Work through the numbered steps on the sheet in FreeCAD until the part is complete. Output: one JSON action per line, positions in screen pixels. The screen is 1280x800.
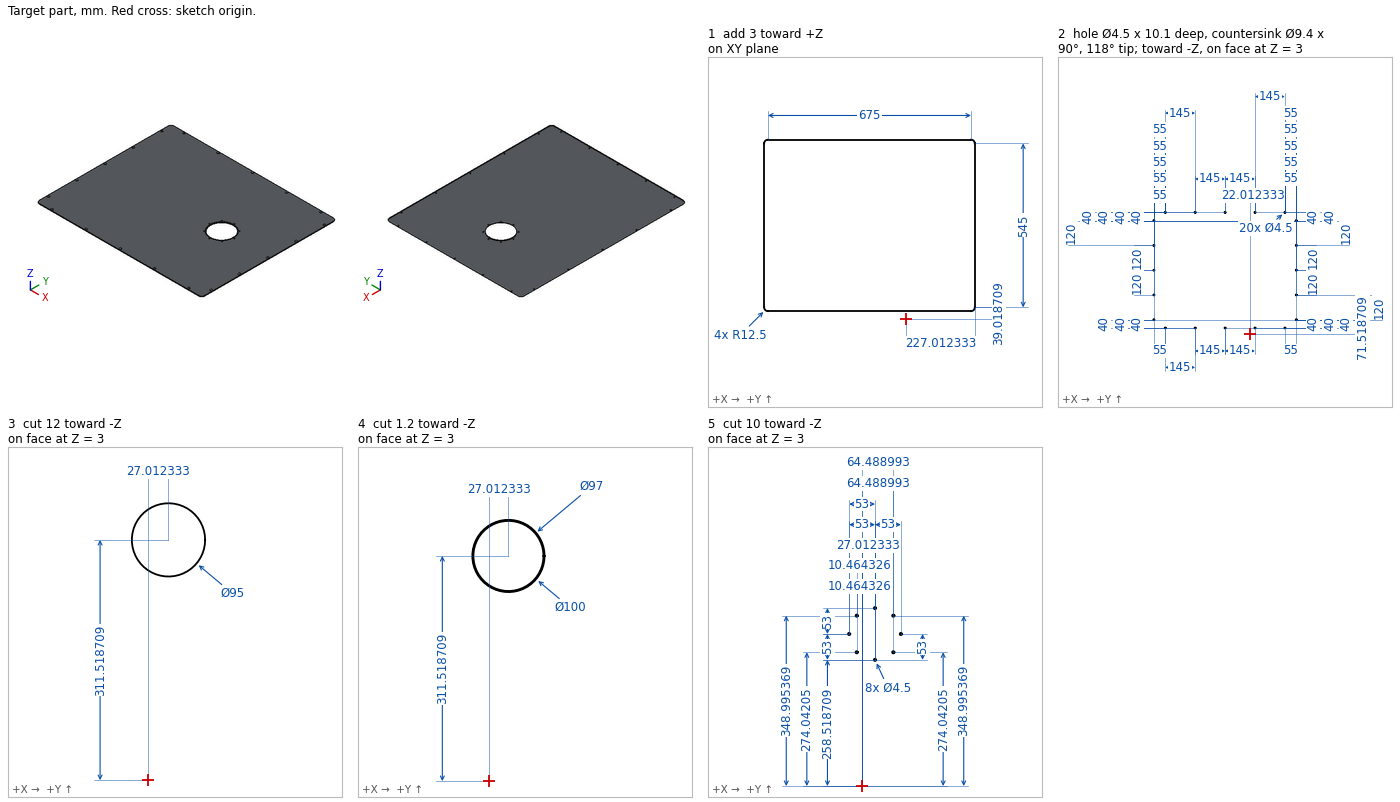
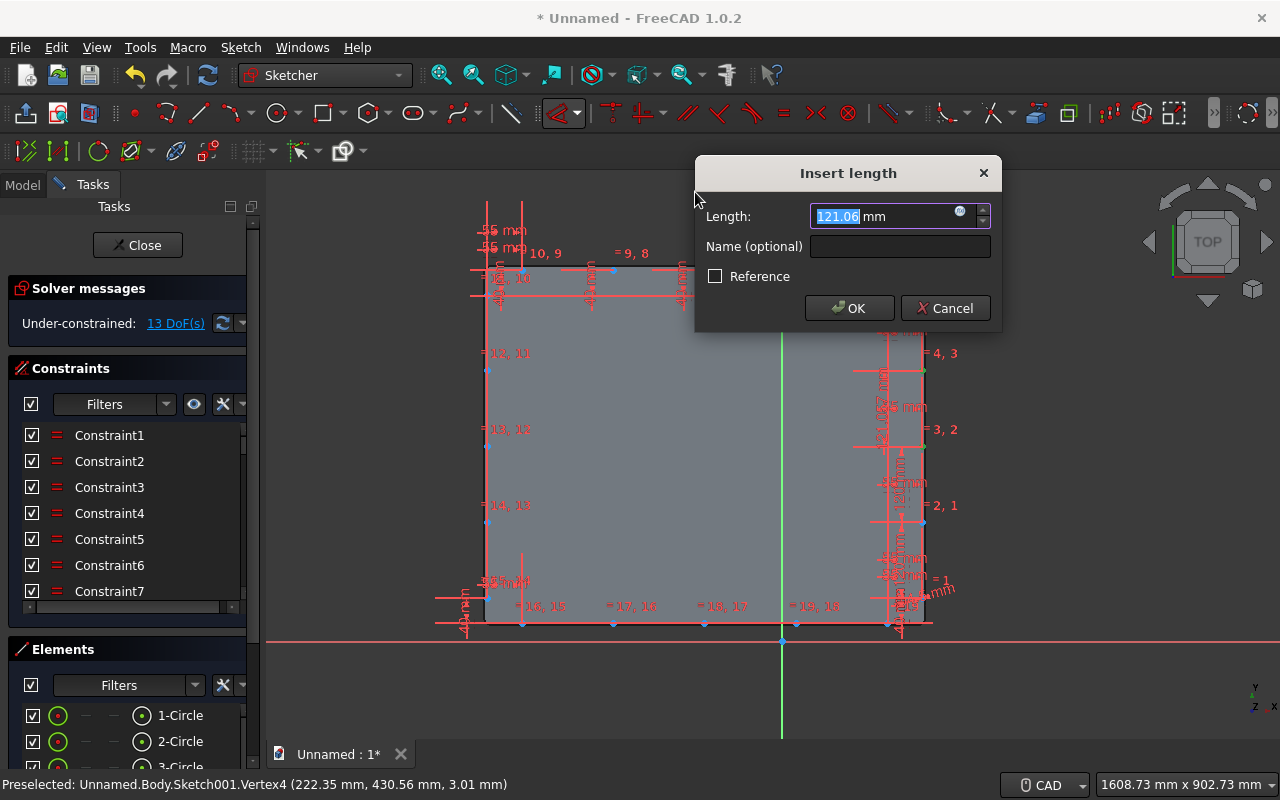
{"action": "type", "text": "120"}
{"action": "key", "text": "Return"}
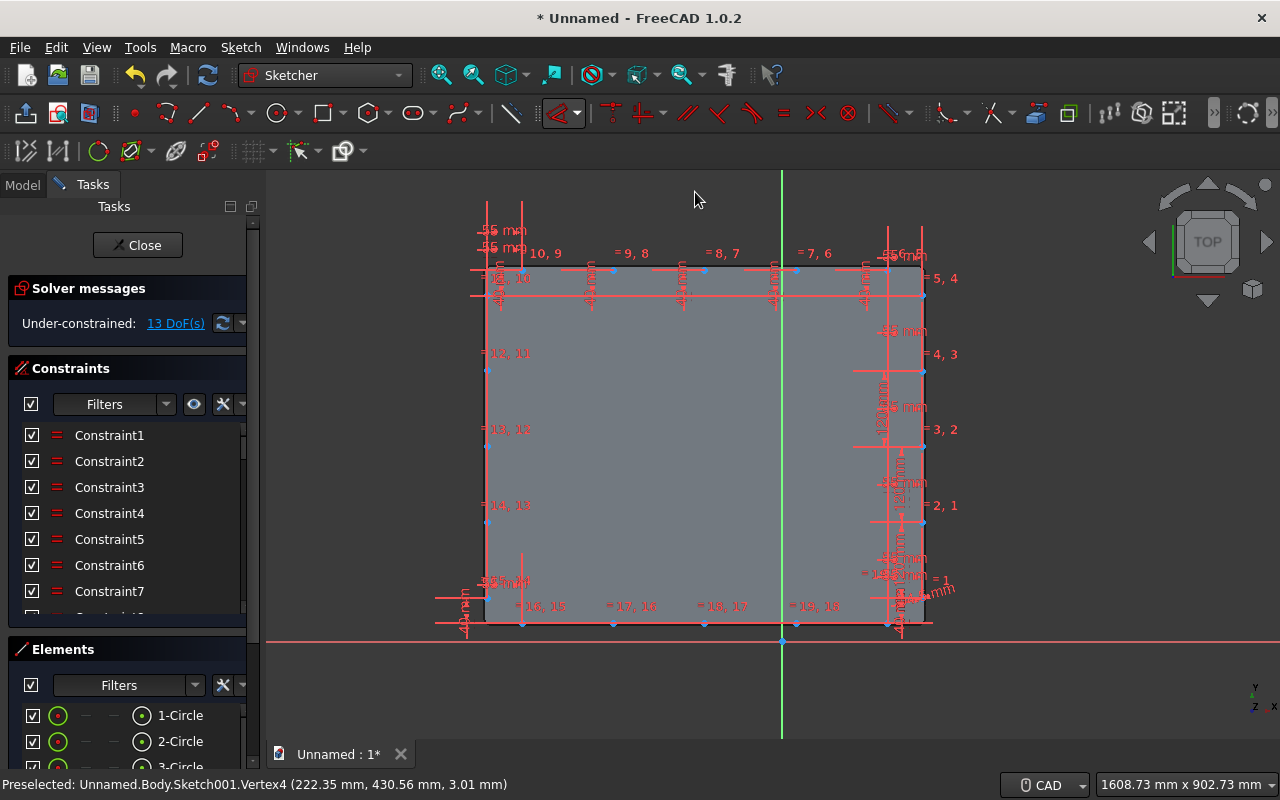
{"action": "left_click", "coordinate": [922, 371]}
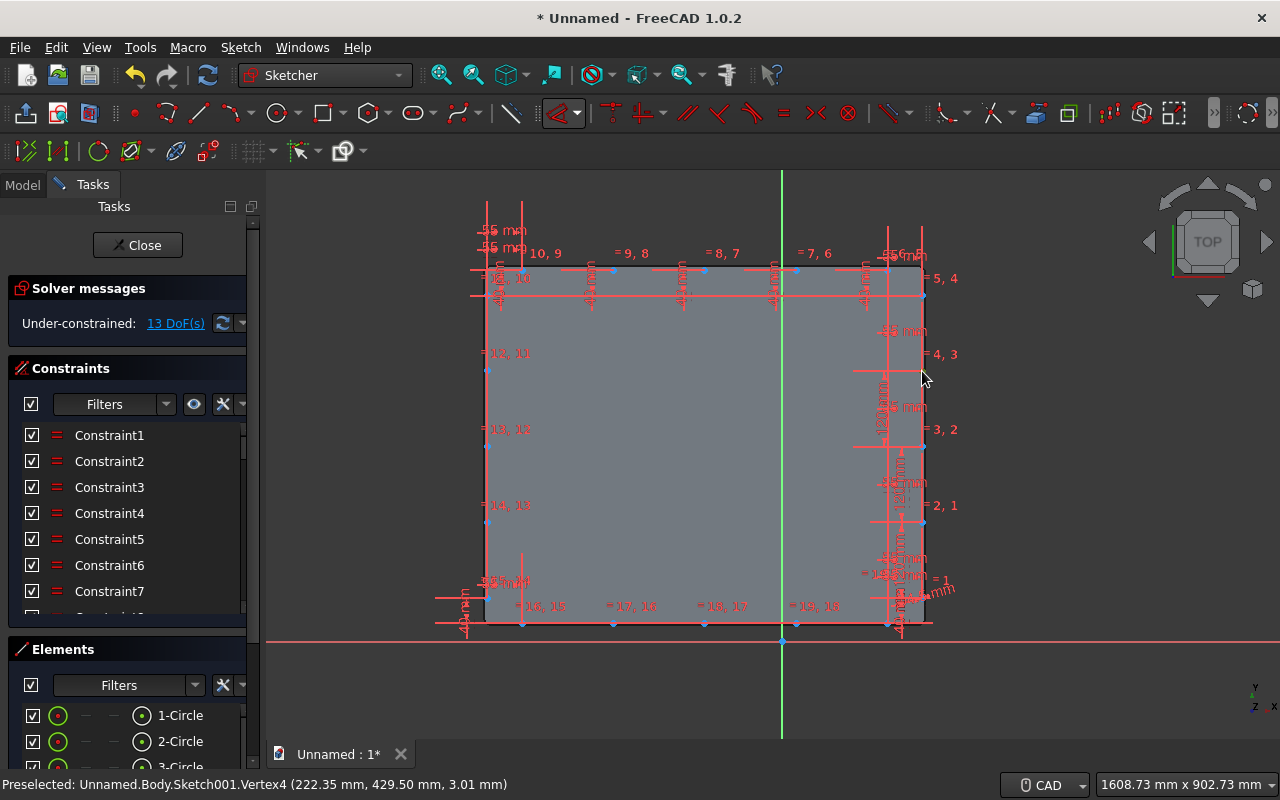
{"action": "left_click", "coordinate": [922, 296]}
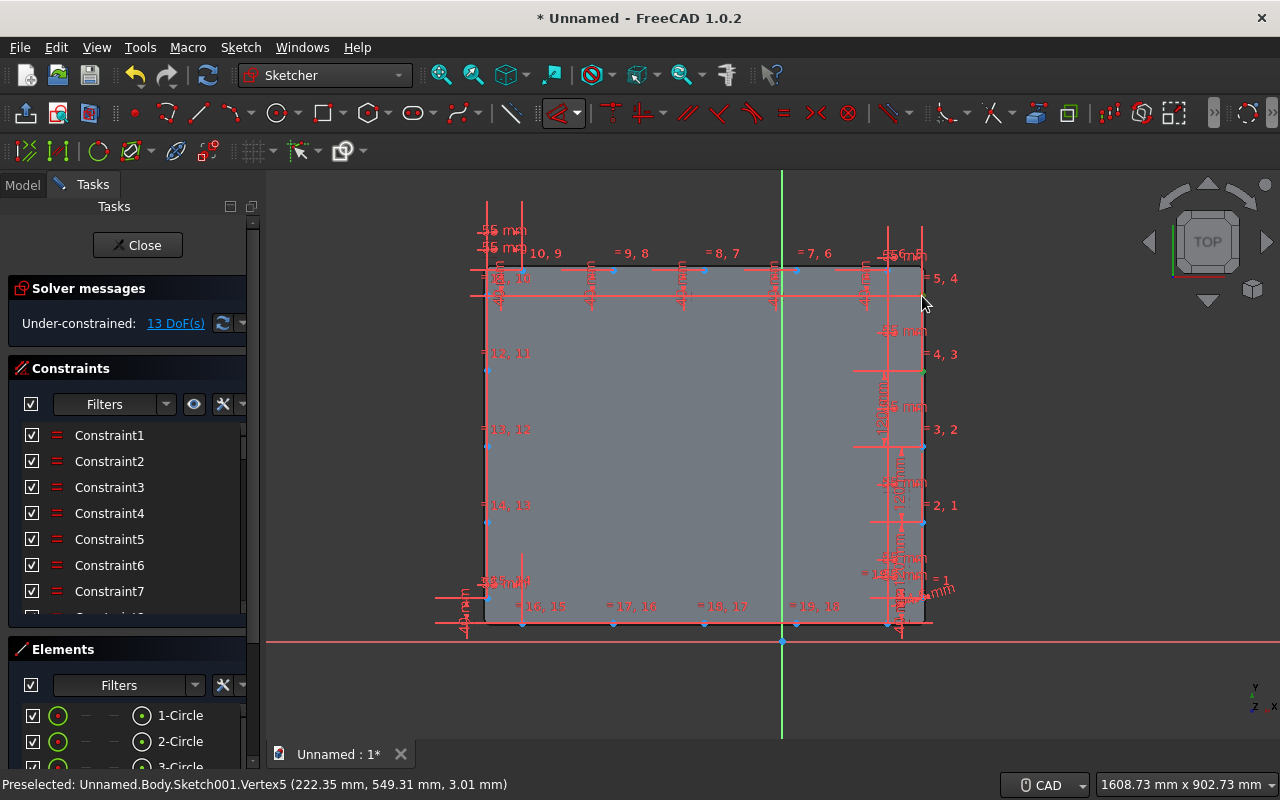
{"action": "key", "text": "i"}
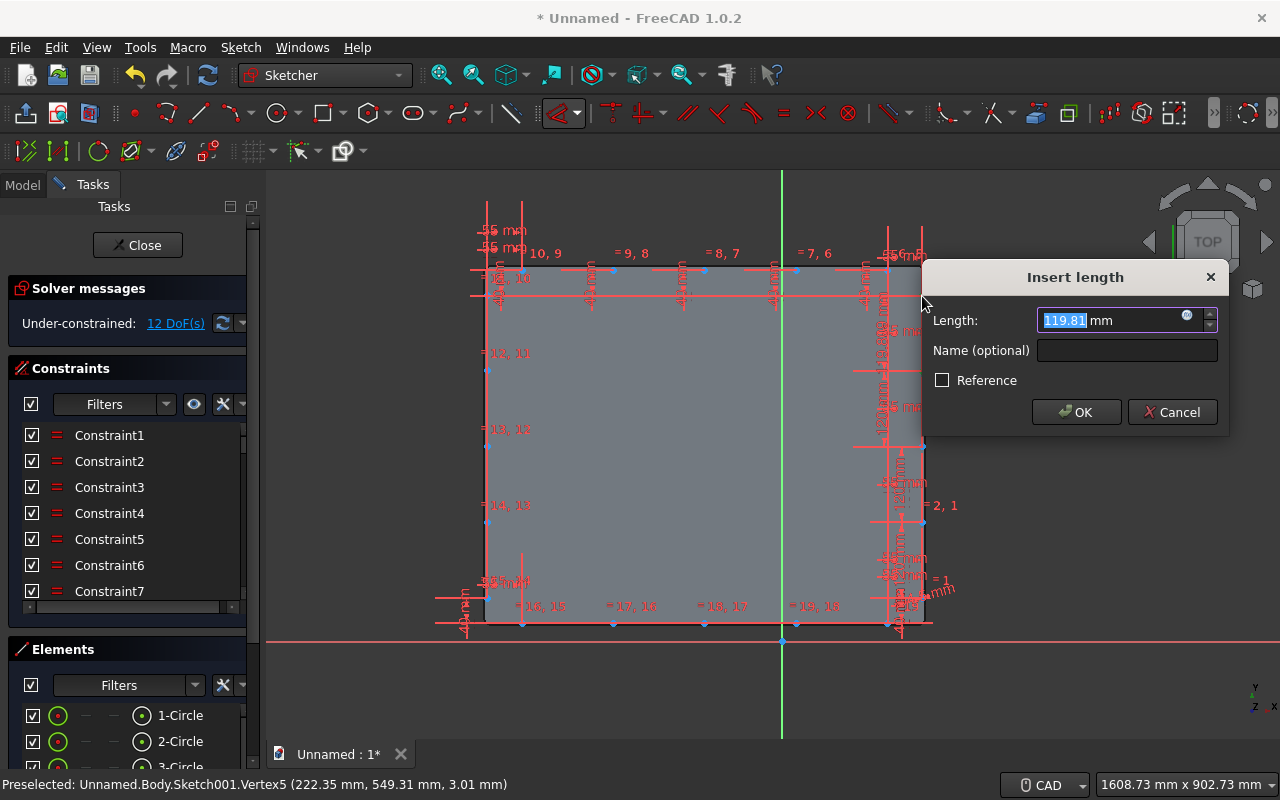
{"action": "type", "text": "120"}
{"action": "key", "text": "Return"}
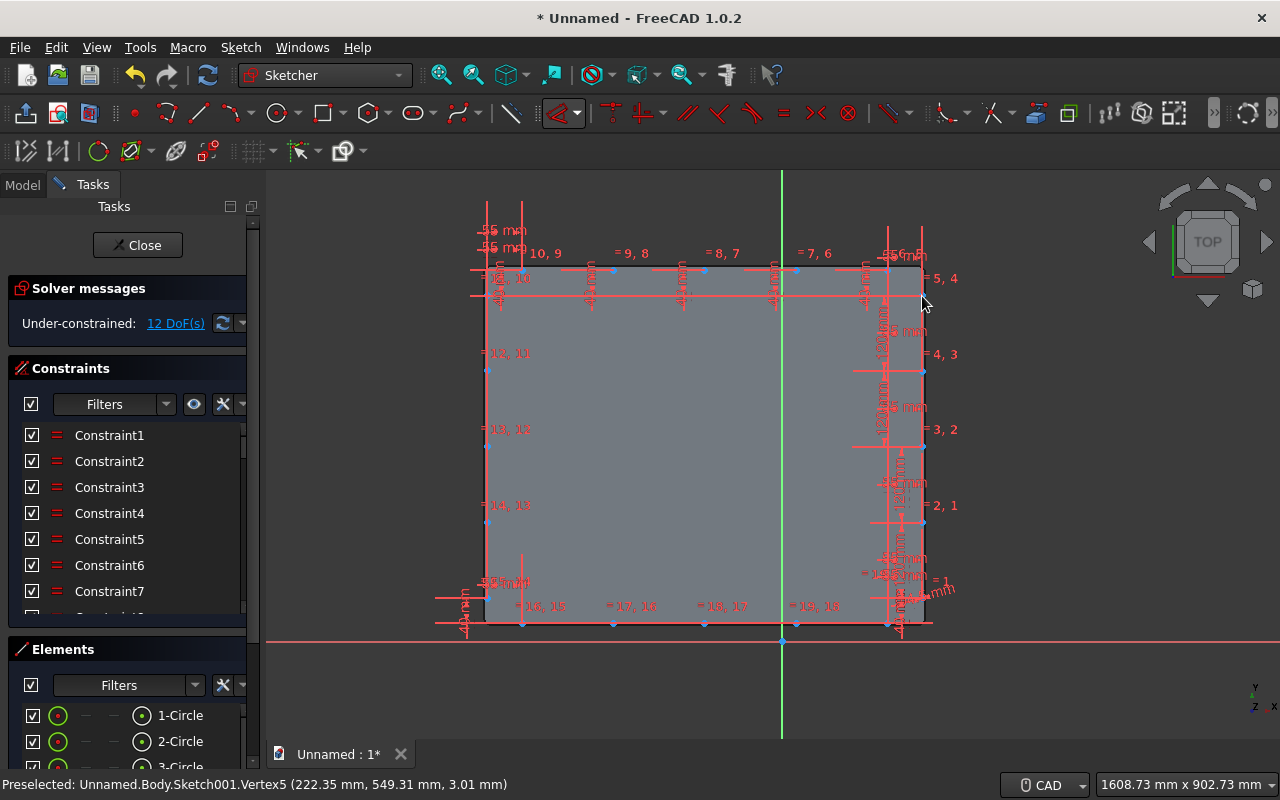
{"action": "left_click", "coordinate": [888, 270]}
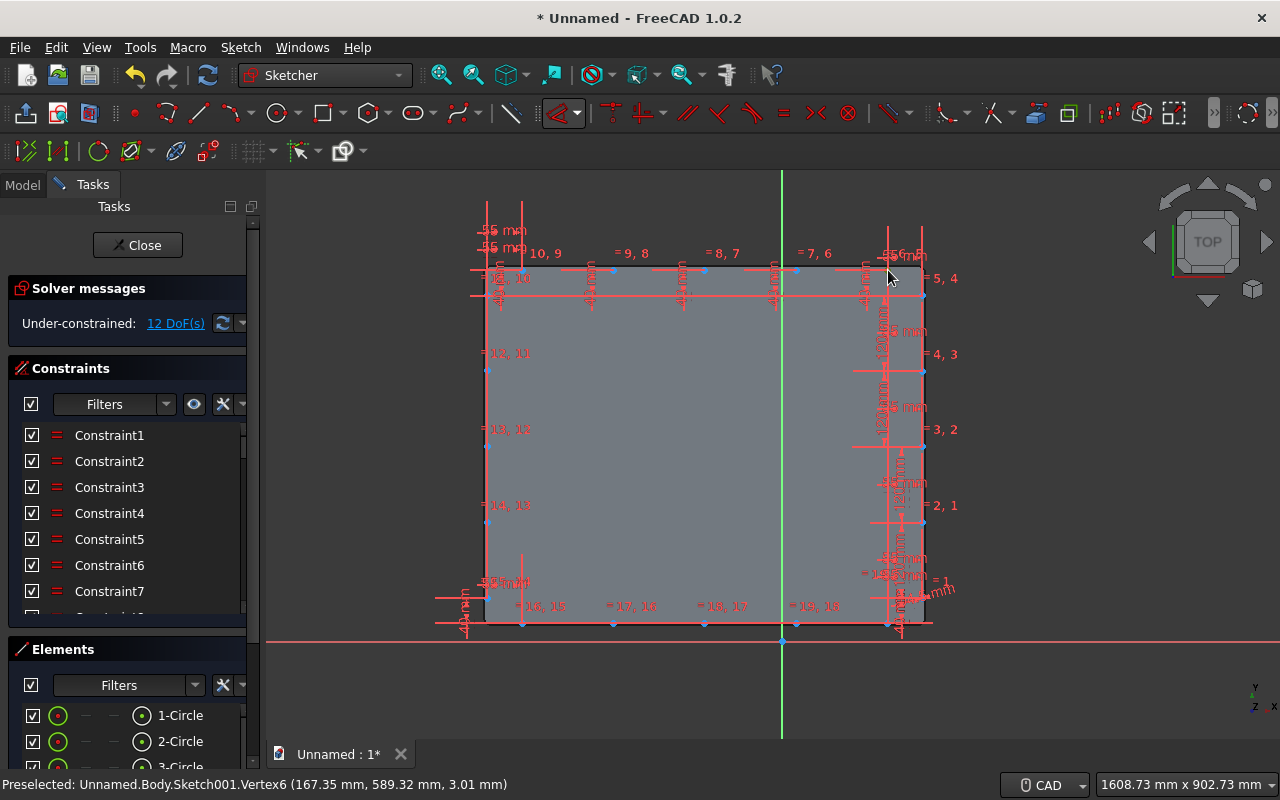
{"action": "left_click", "coordinate": [796, 270]}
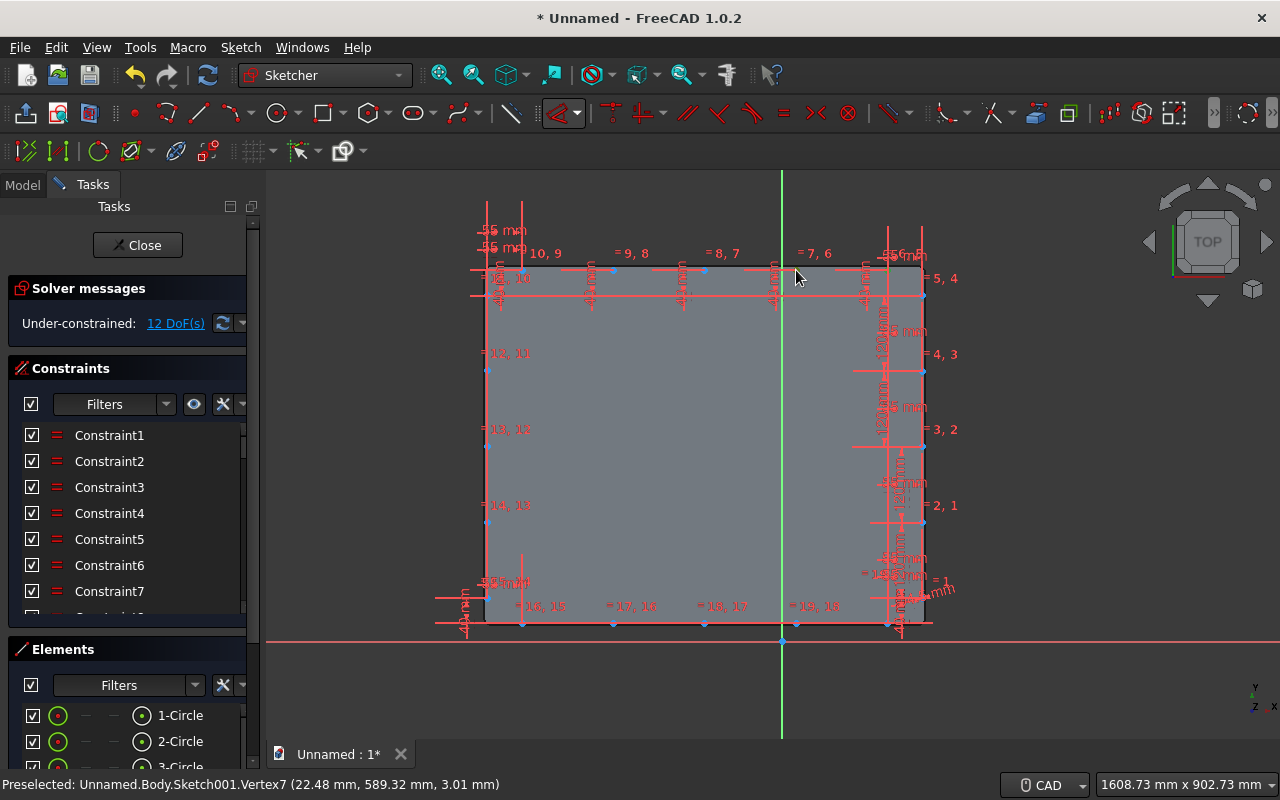
{"action": "key", "text": "l"}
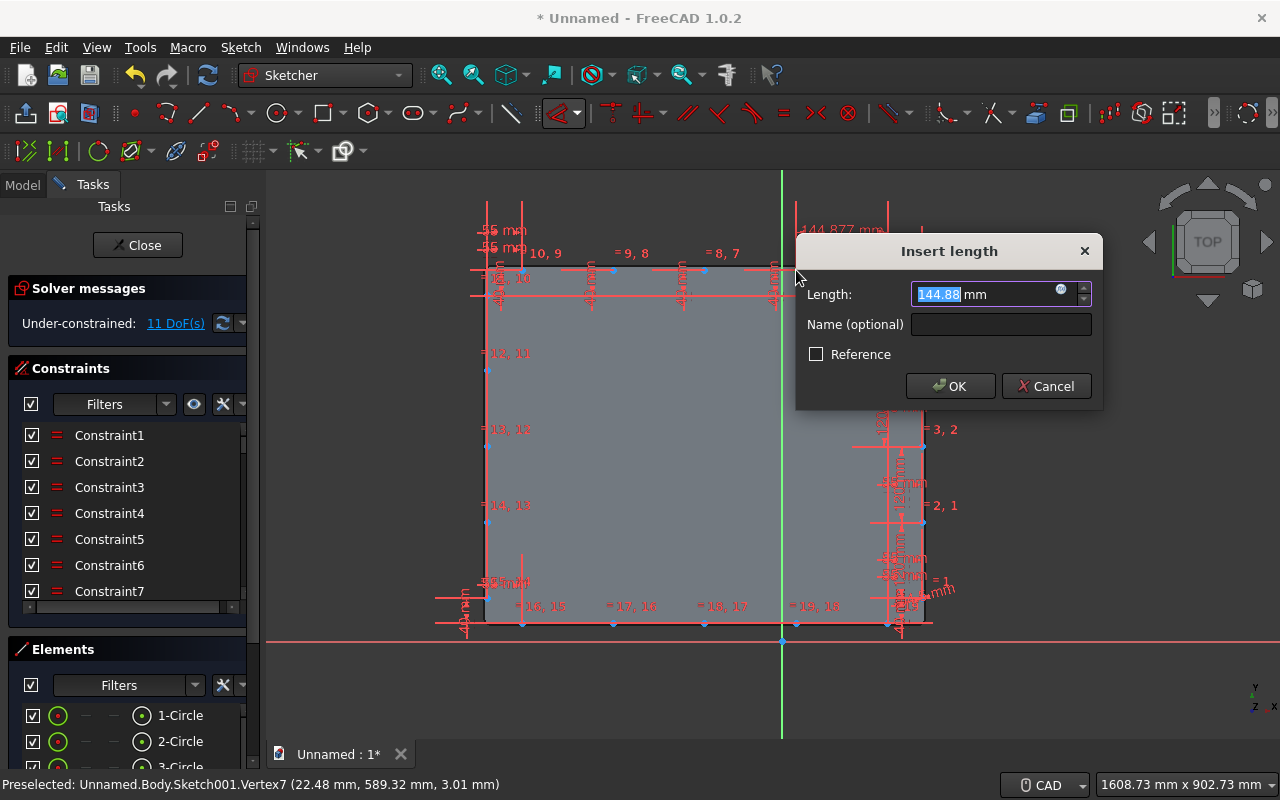
{"action": "type", "text": "145"}
{"action": "key", "text": "Return"}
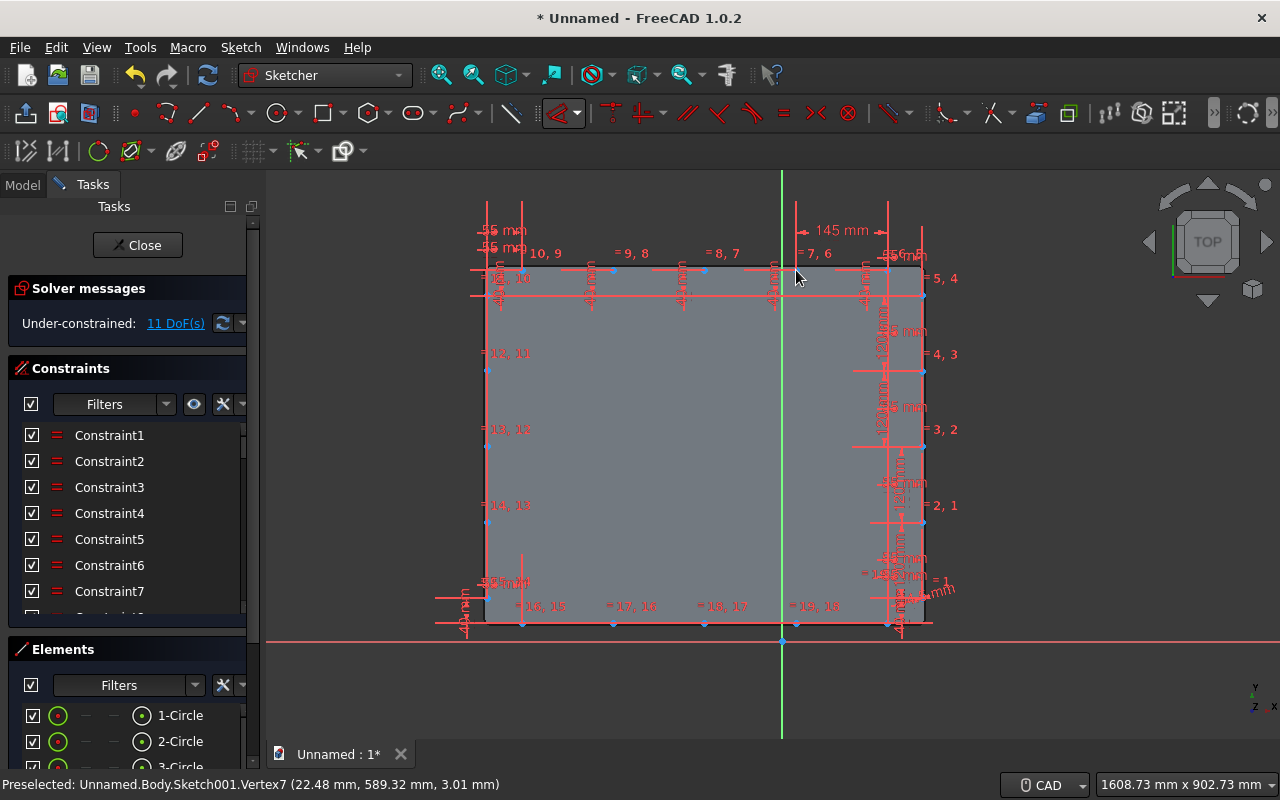
{"action": "left_click", "coordinate": [796, 270]}